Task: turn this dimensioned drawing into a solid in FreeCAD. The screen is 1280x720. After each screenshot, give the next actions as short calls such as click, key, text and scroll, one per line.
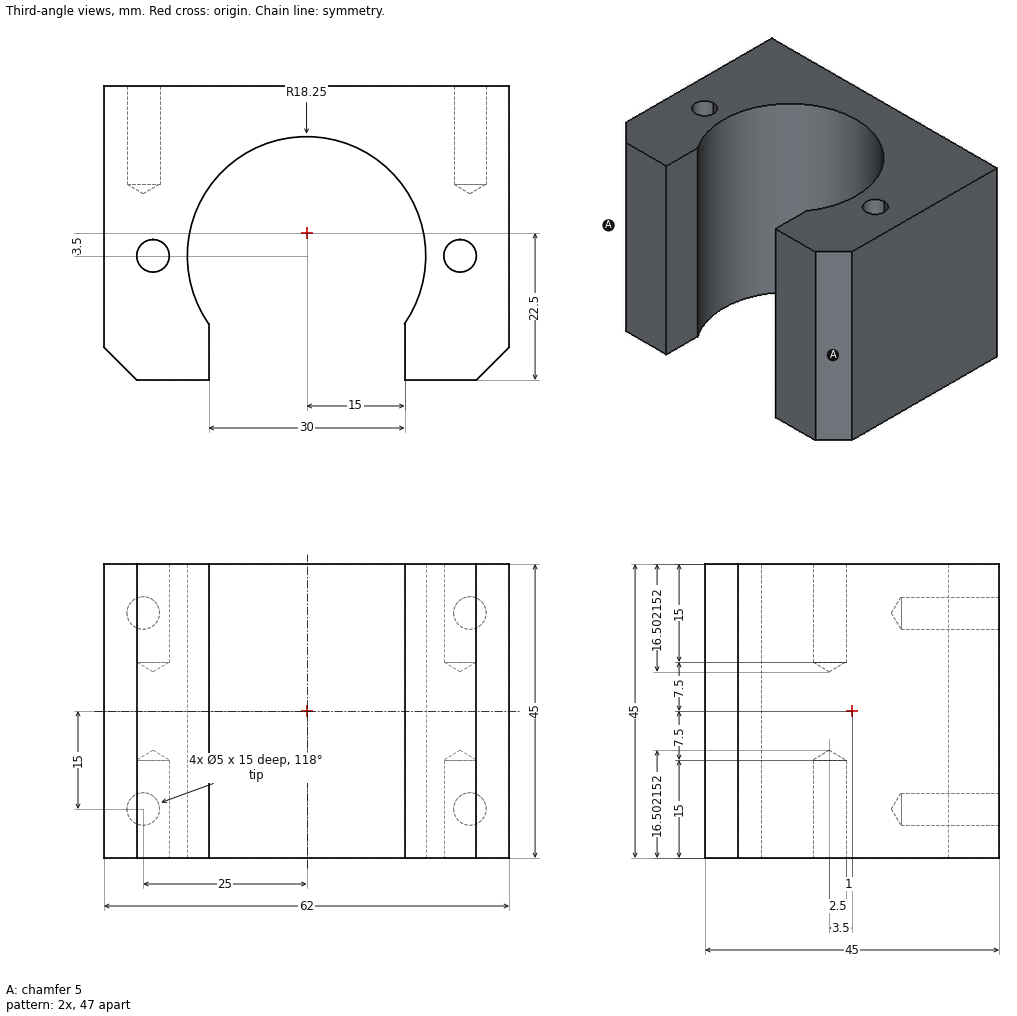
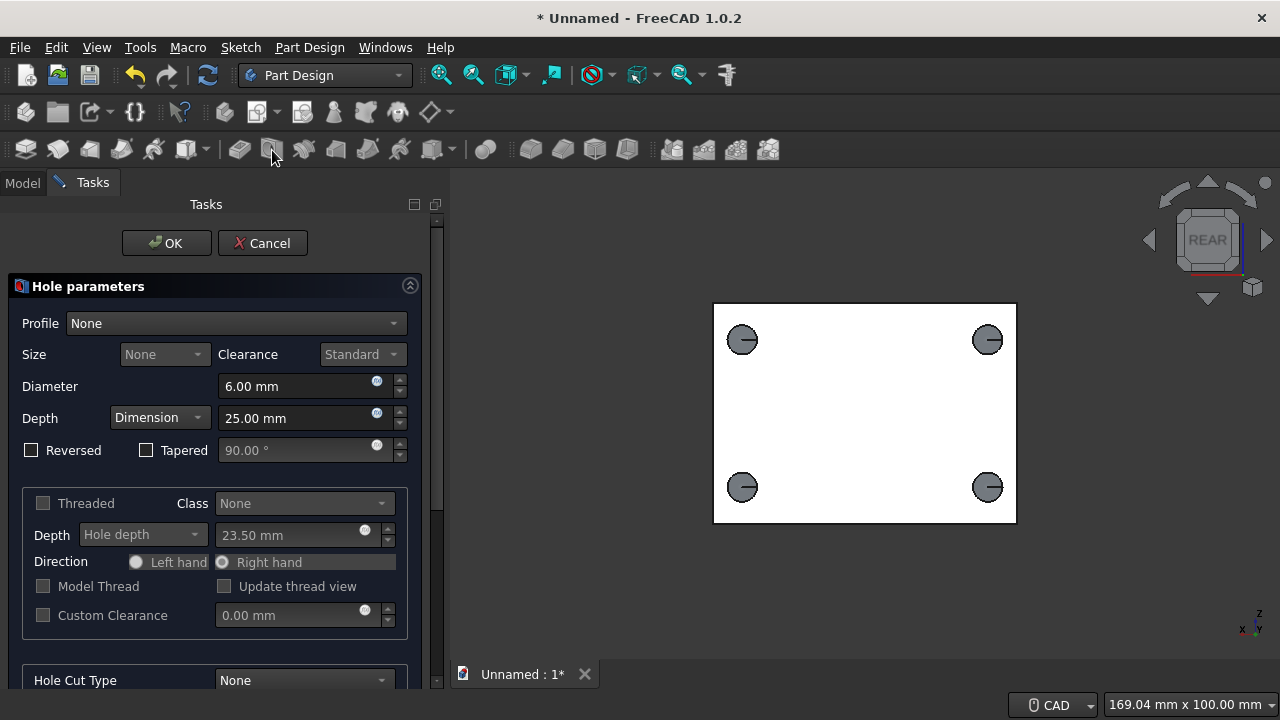
triple_click(305, 386)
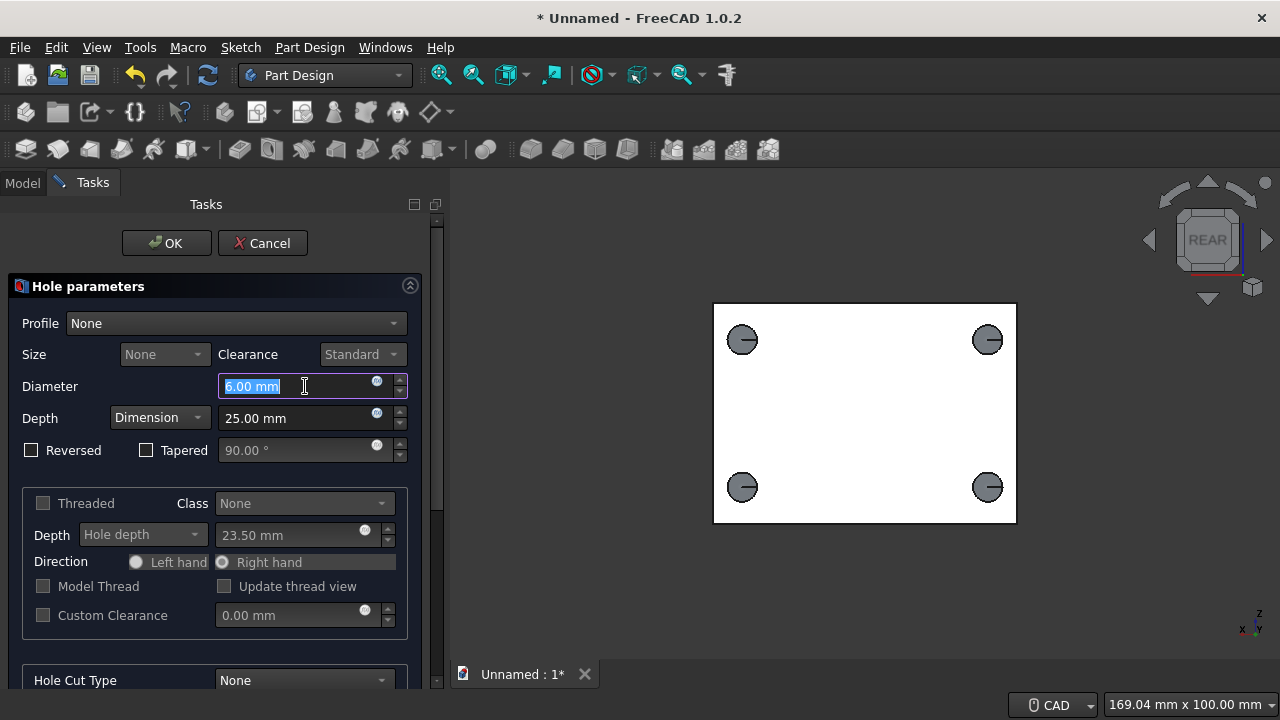
text(5)
key(Tab)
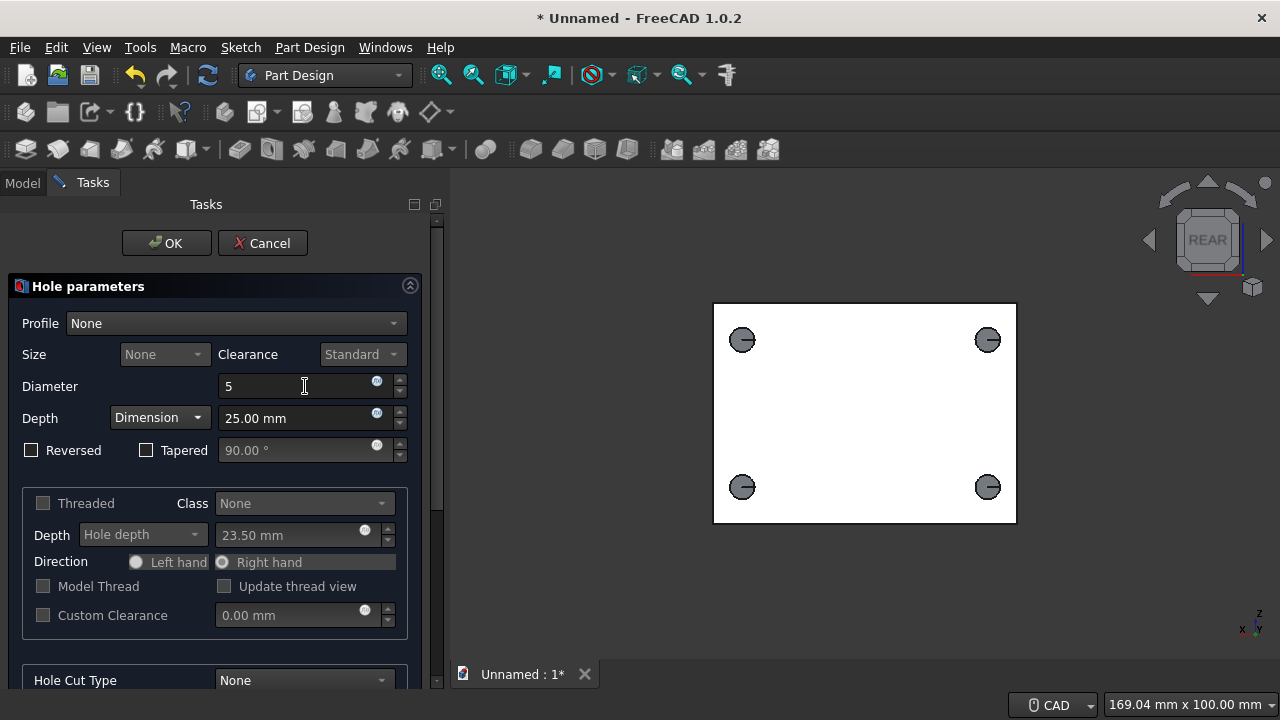
triple_click(305, 418)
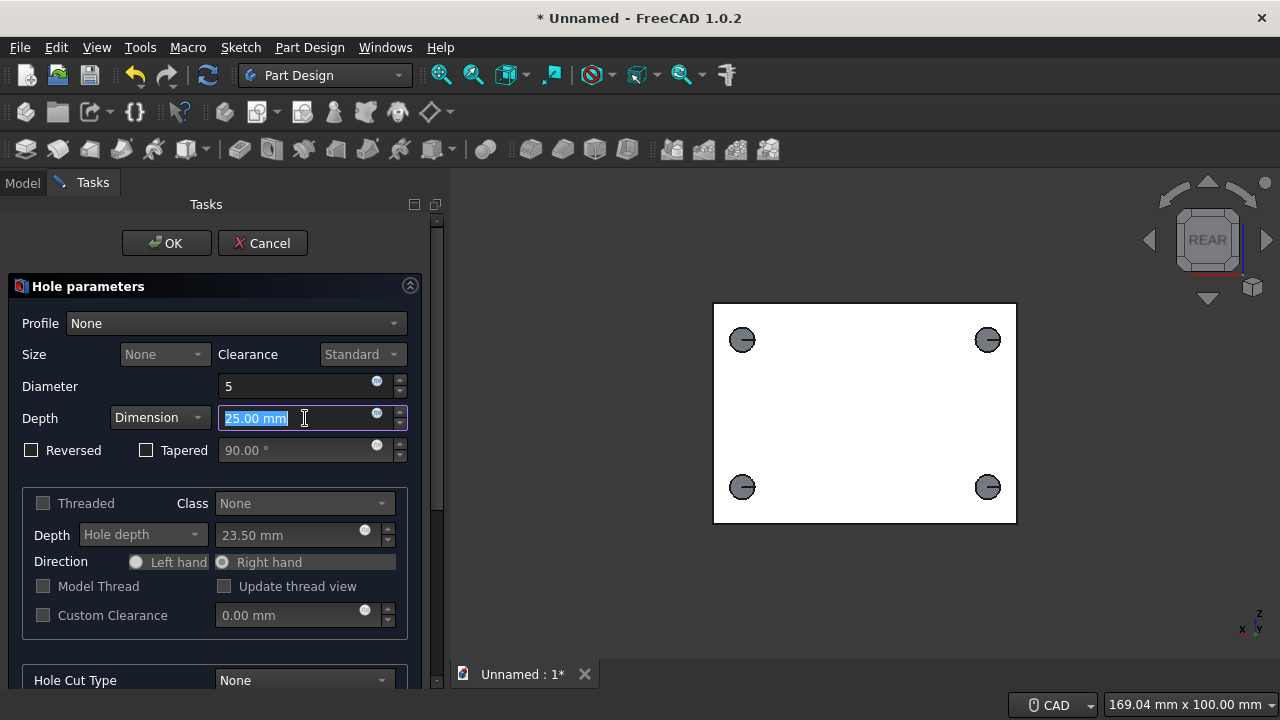
text(15)
key(Tab)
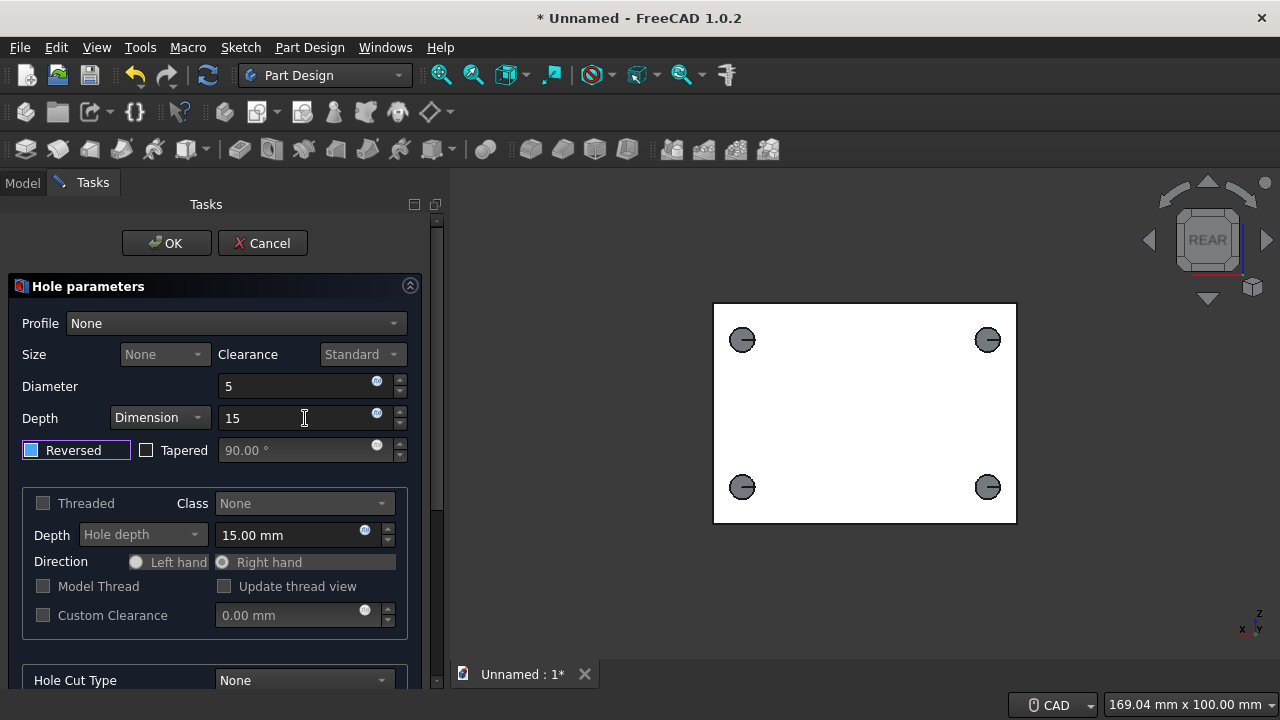
click(167, 243)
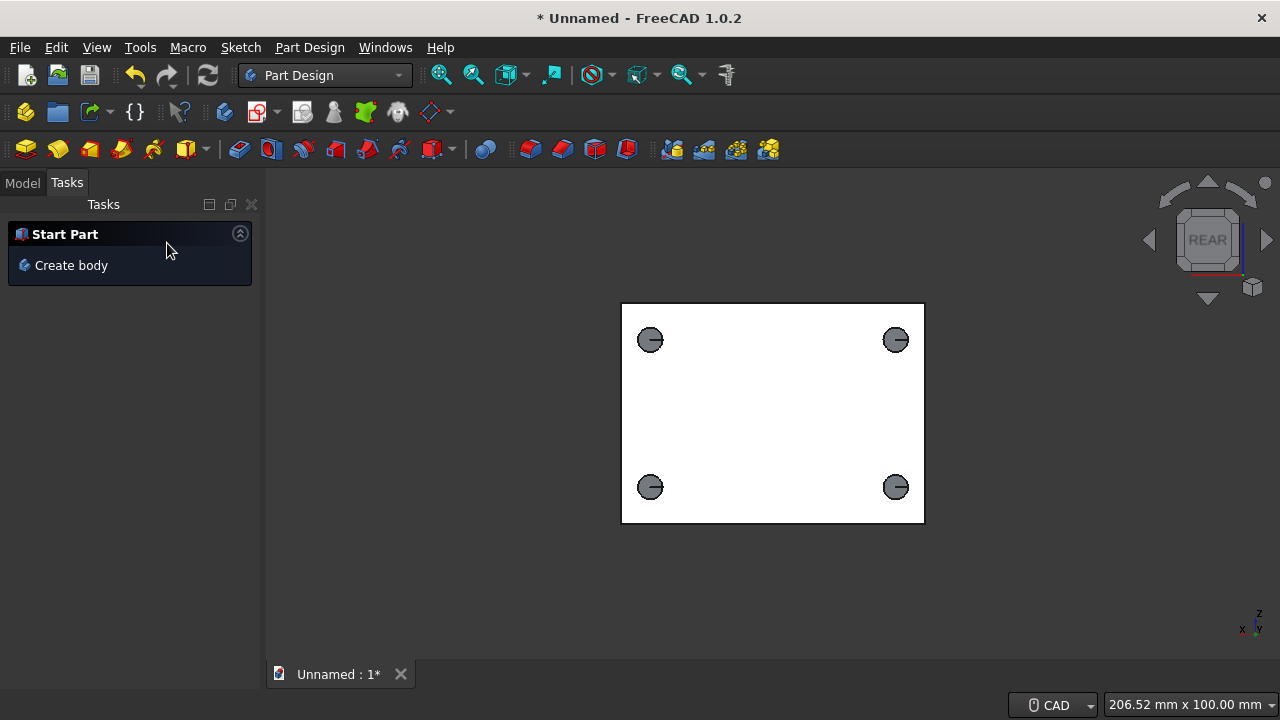
click(23, 182)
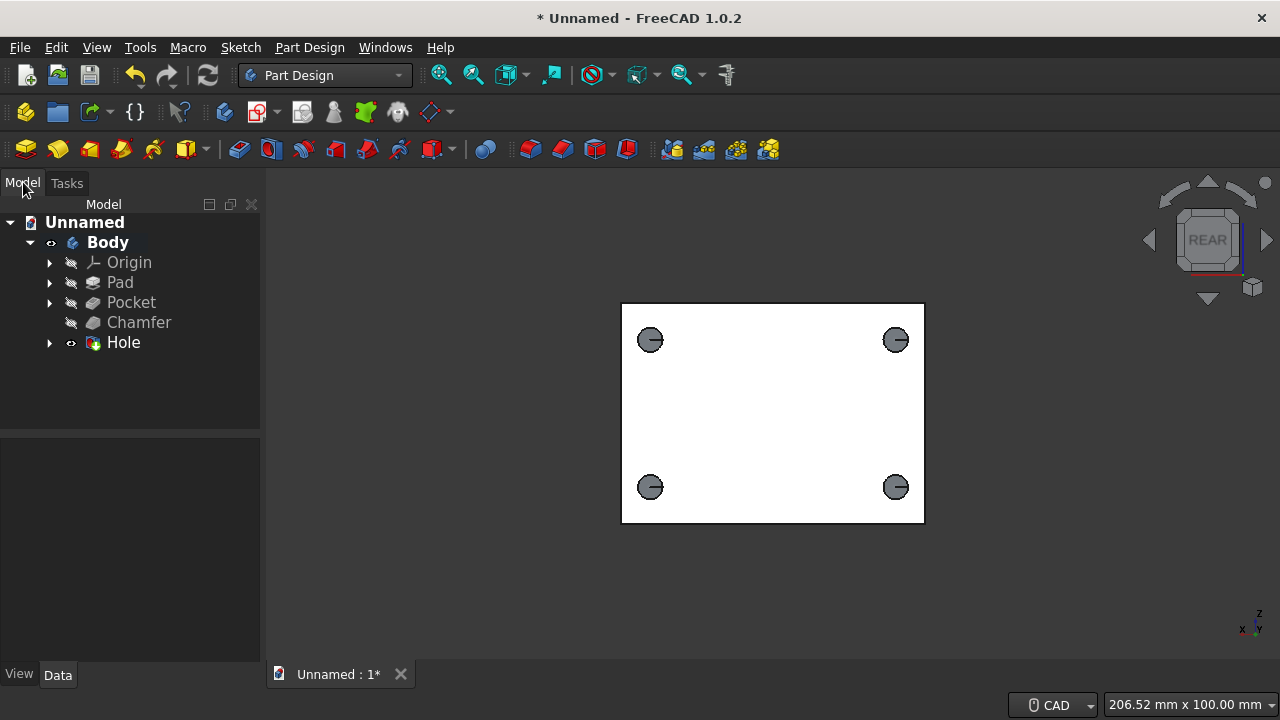
click(50, 263)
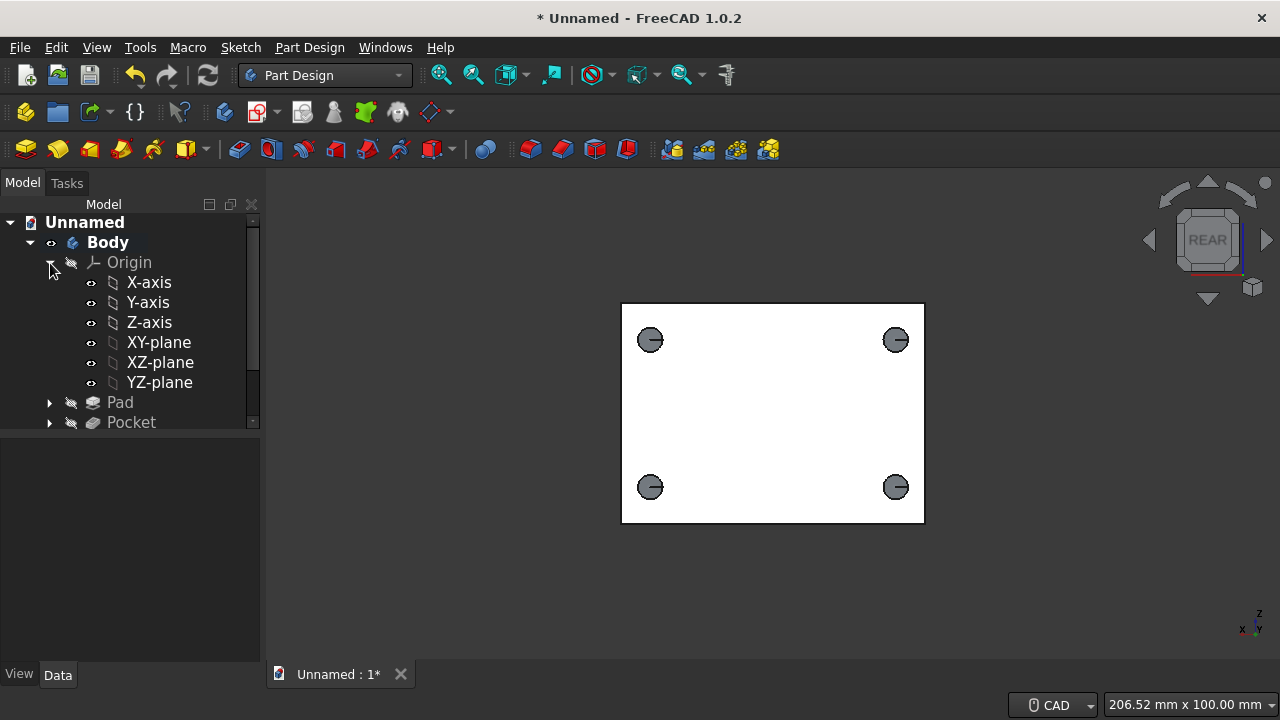
click(136, 383)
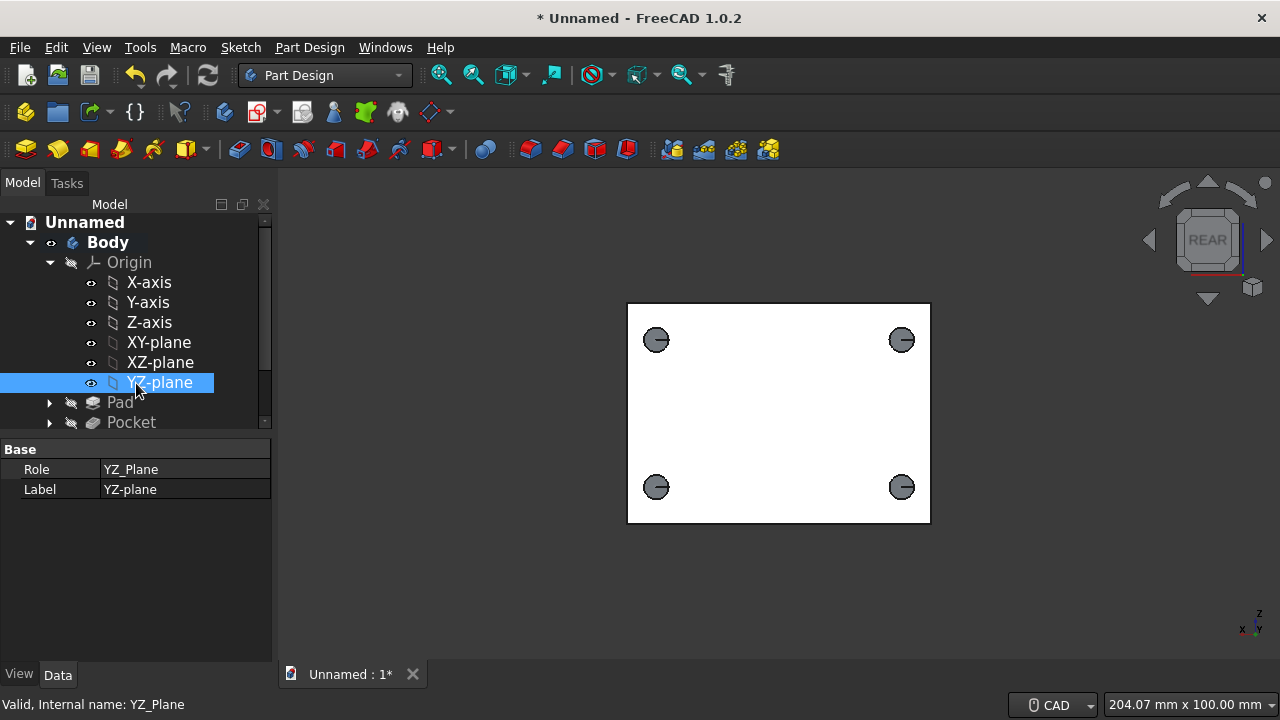
click(430, 112)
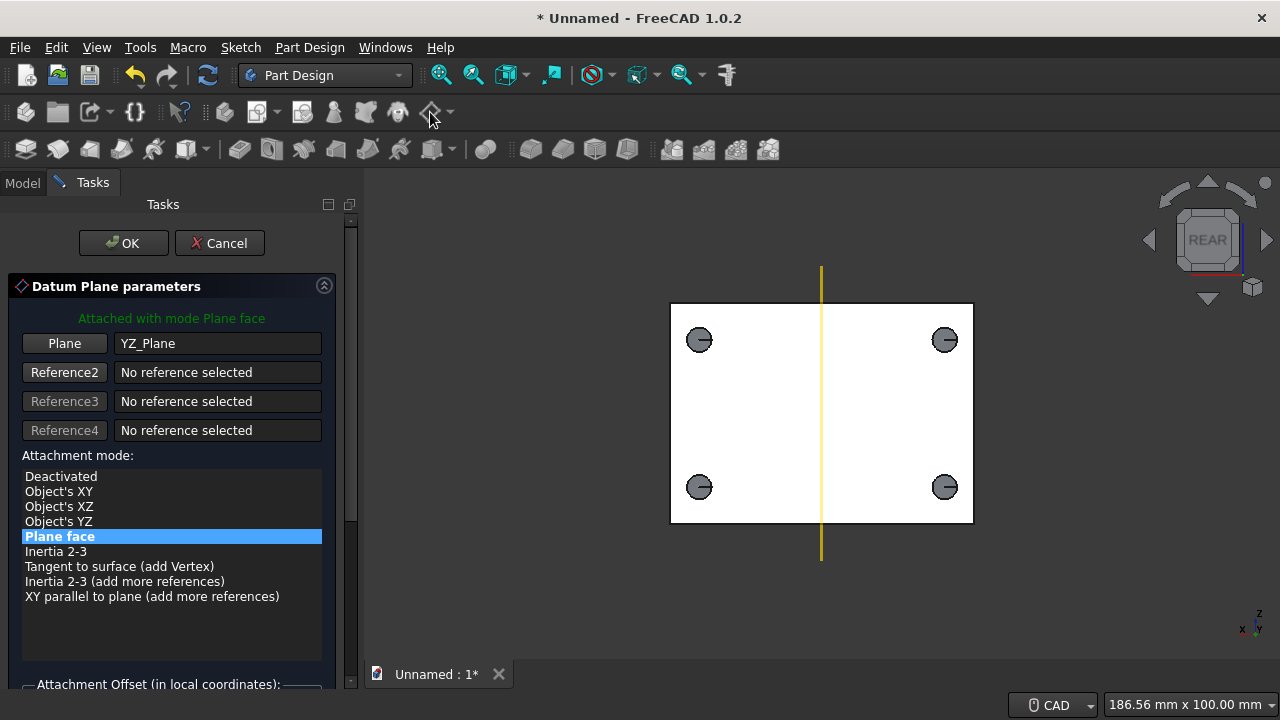
scroll(351, 451, down, 3)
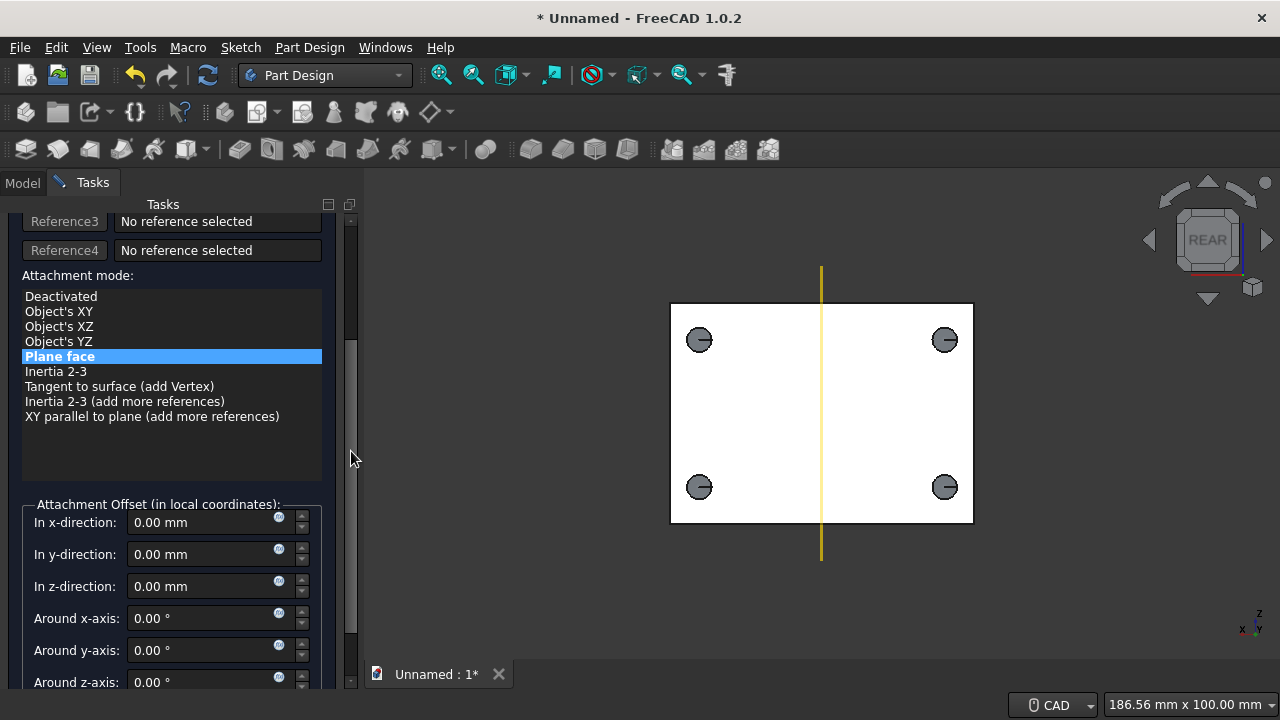
triple_click(210, 586)